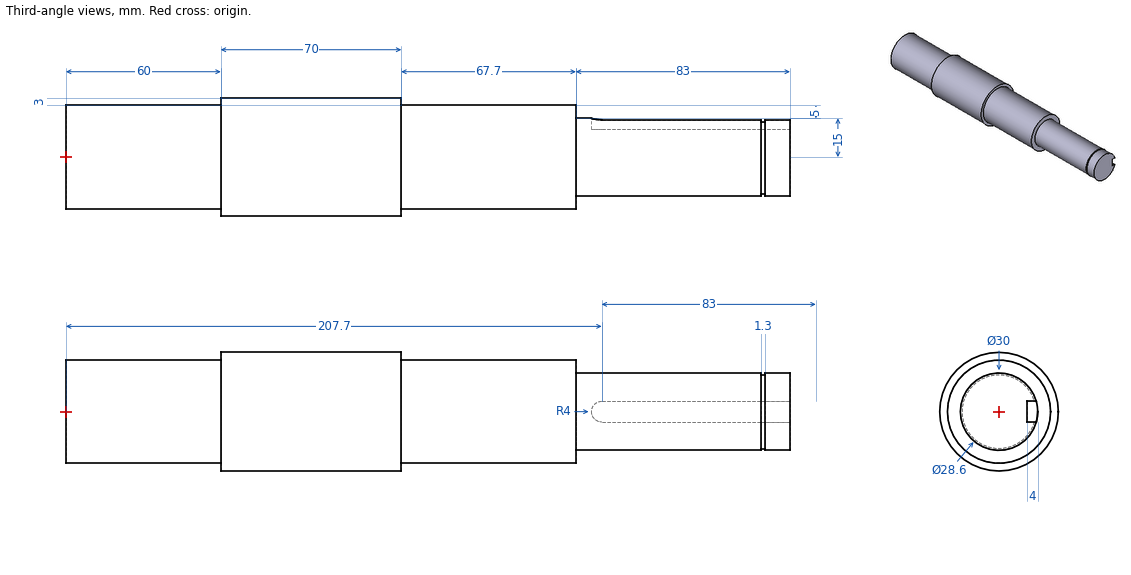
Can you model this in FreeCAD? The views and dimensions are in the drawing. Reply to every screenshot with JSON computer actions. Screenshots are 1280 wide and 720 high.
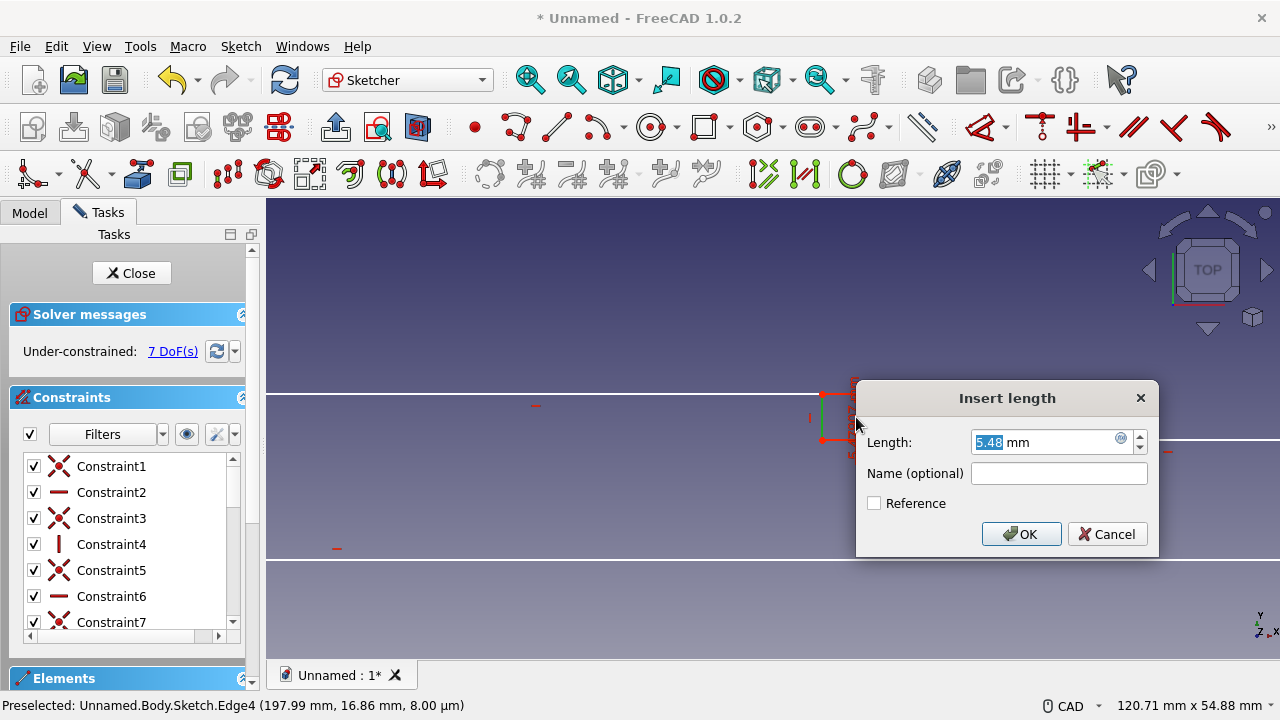
{"action": "type", "text": "5"}
{"action": "key", "text": "Return"}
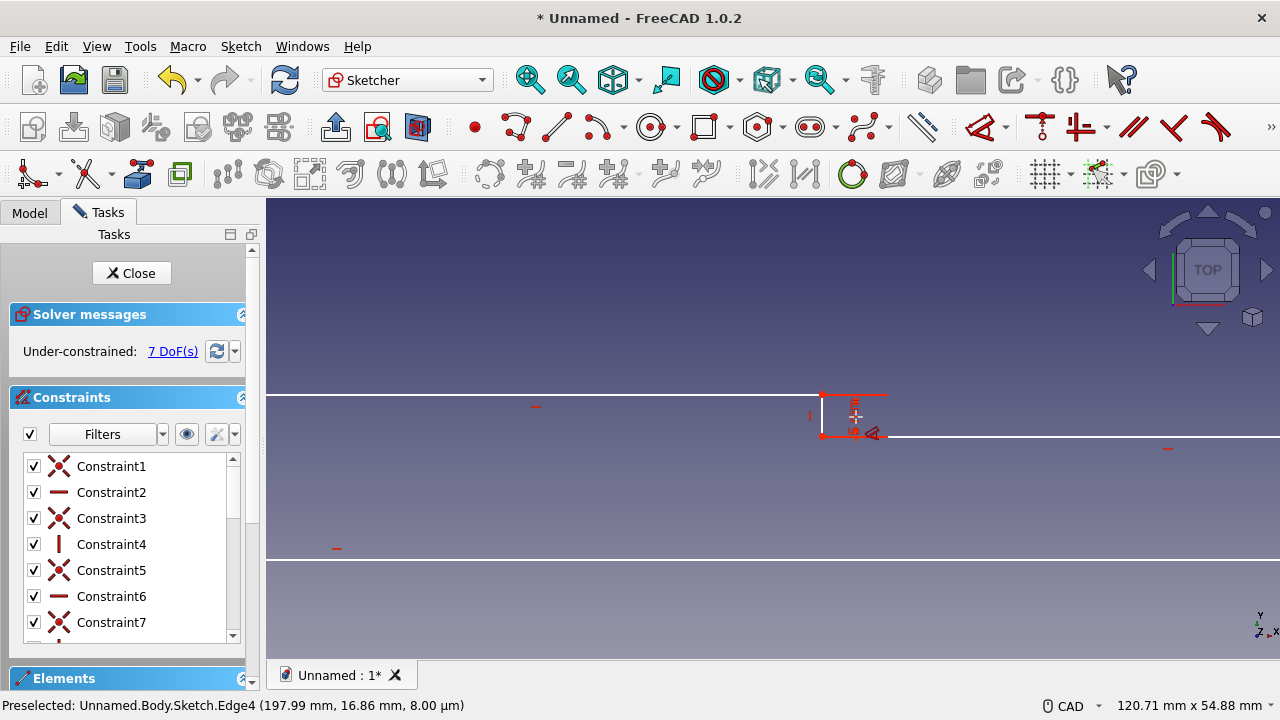
{"action": "scroll", "coordinate": [824, 417], "scroll_direction": "down", "scroll_amount": 7}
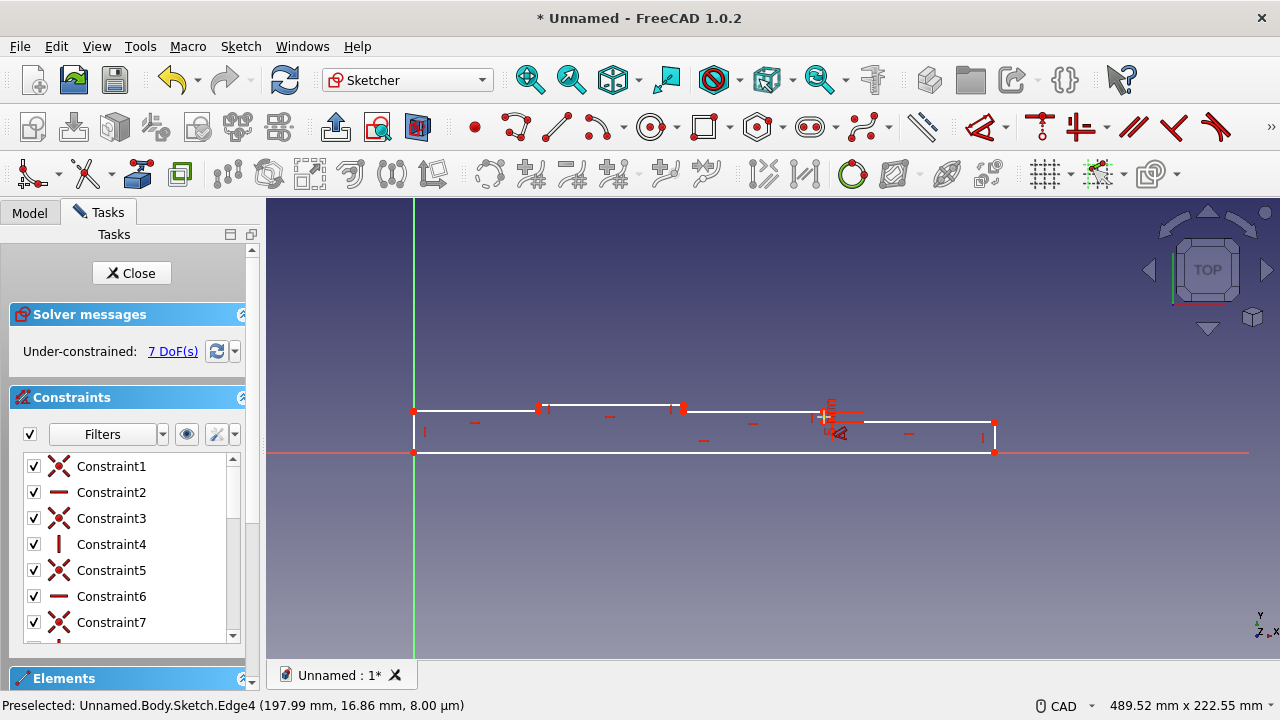
{"action": "scroll", "coordinate": [683, 409], "scroll_direction": "up", "scroll_amount": 10}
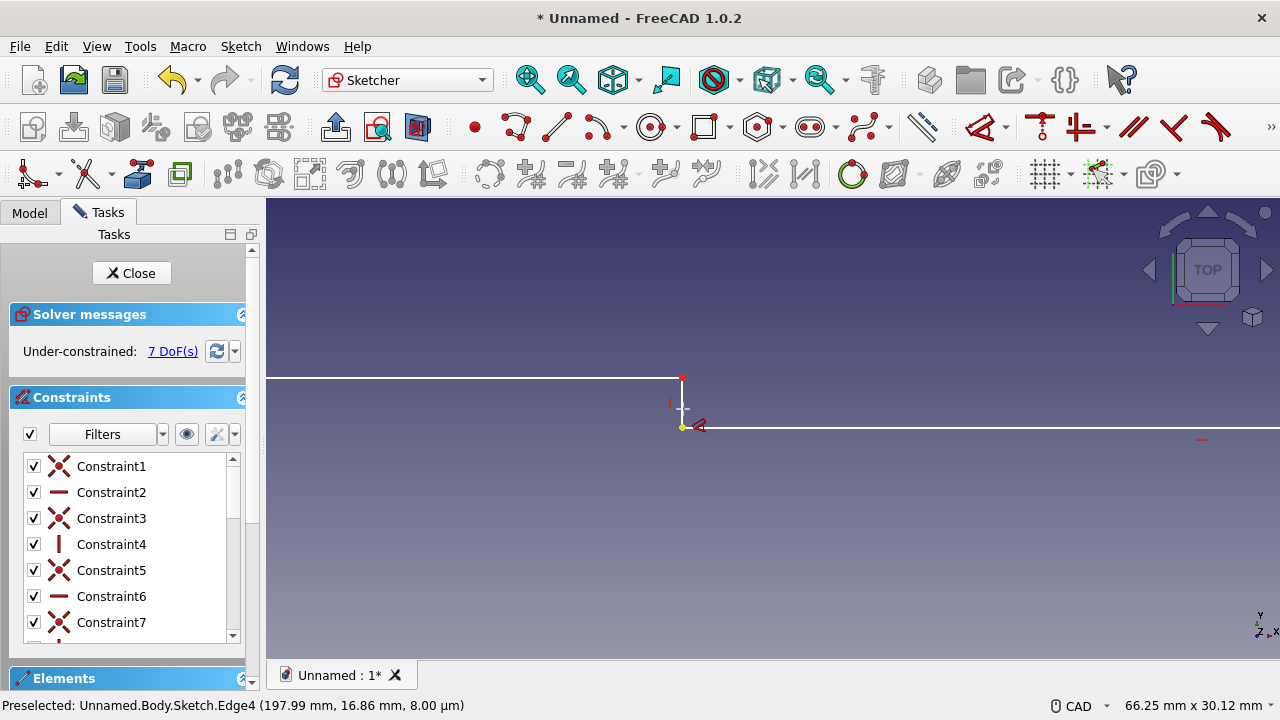
{"action": "left_click", "coordinate": [682, 408]}
{"action": "left_click", "coordinate": [648, 403]}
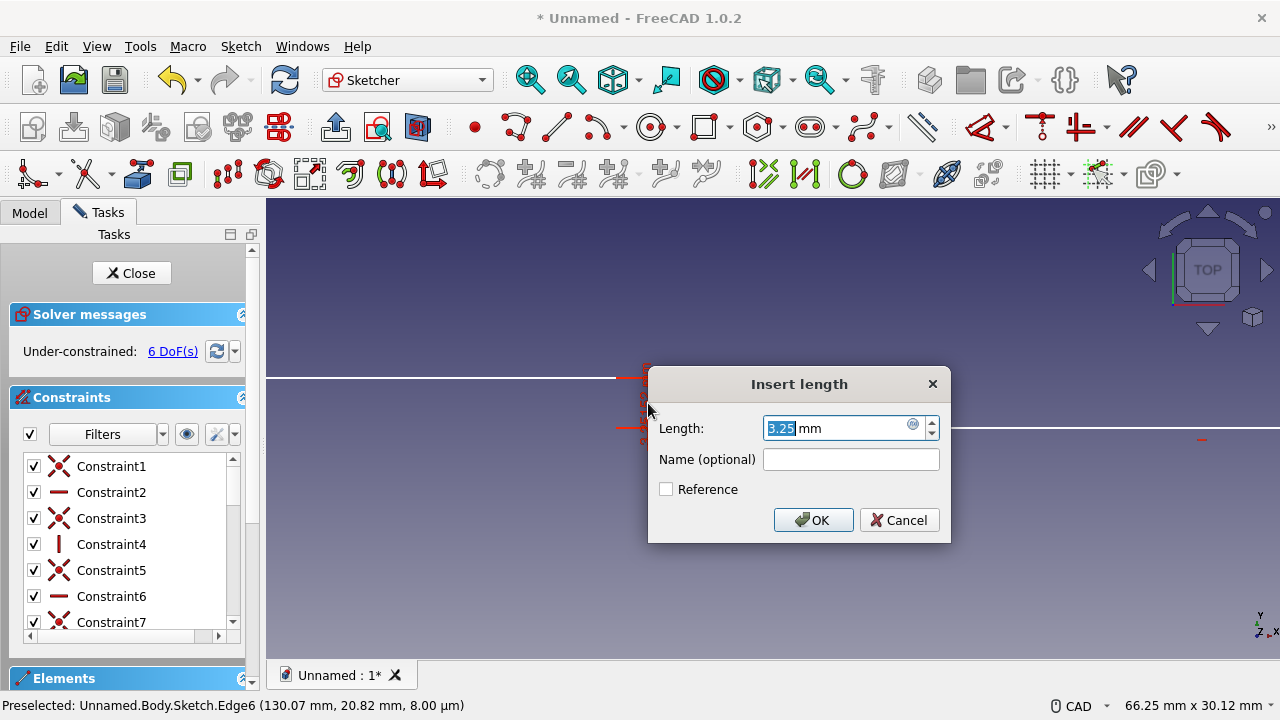
{"action": "type", "text": "3"}
{"action": "key", "text": "Return"}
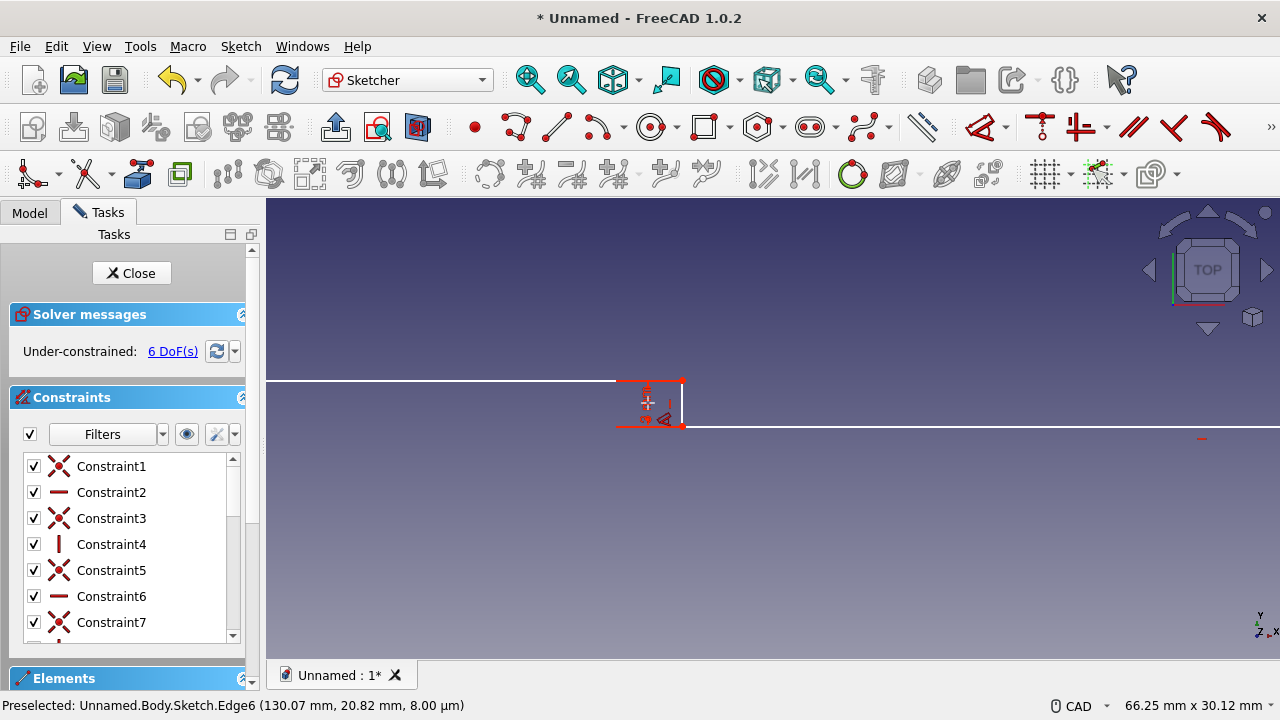
{"action": "scroll", "coordinate": [683, 409], "scroll_direction": "down", "scroll_amount": 10}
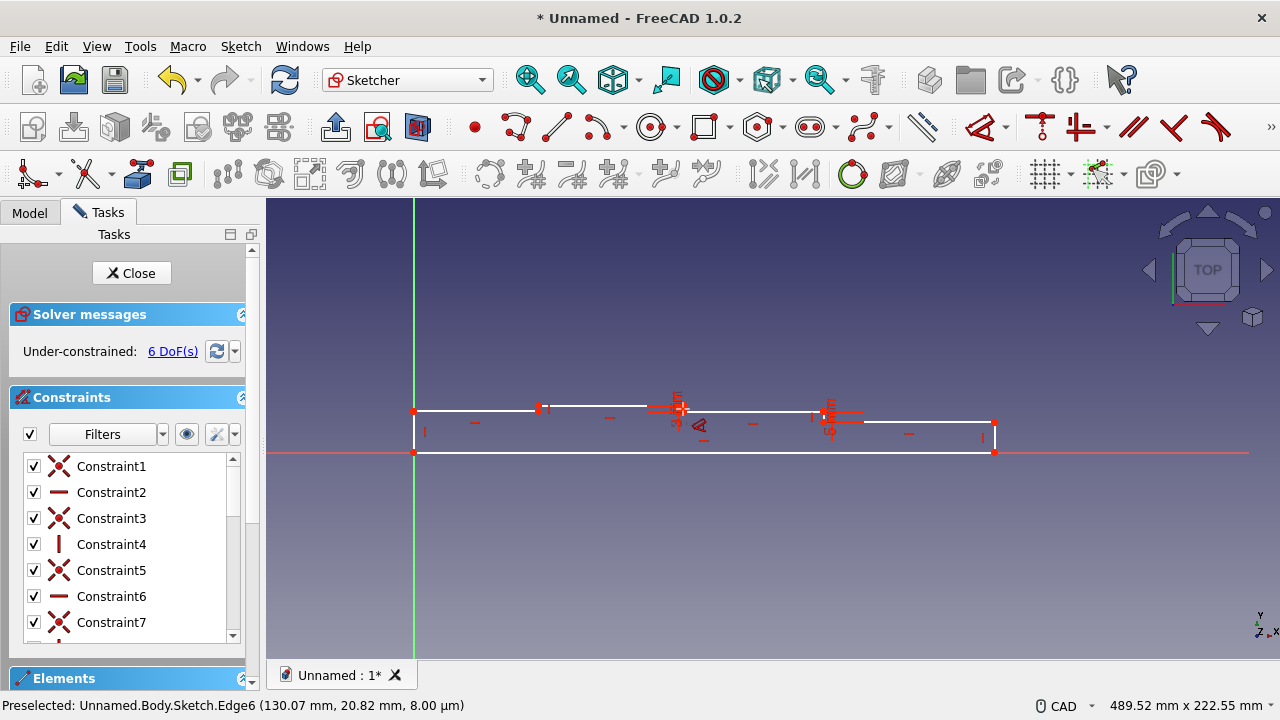
{"action": "scroll", "coordinate": [538, 407], "scroll_direction": "up", "scroll_amount": 11}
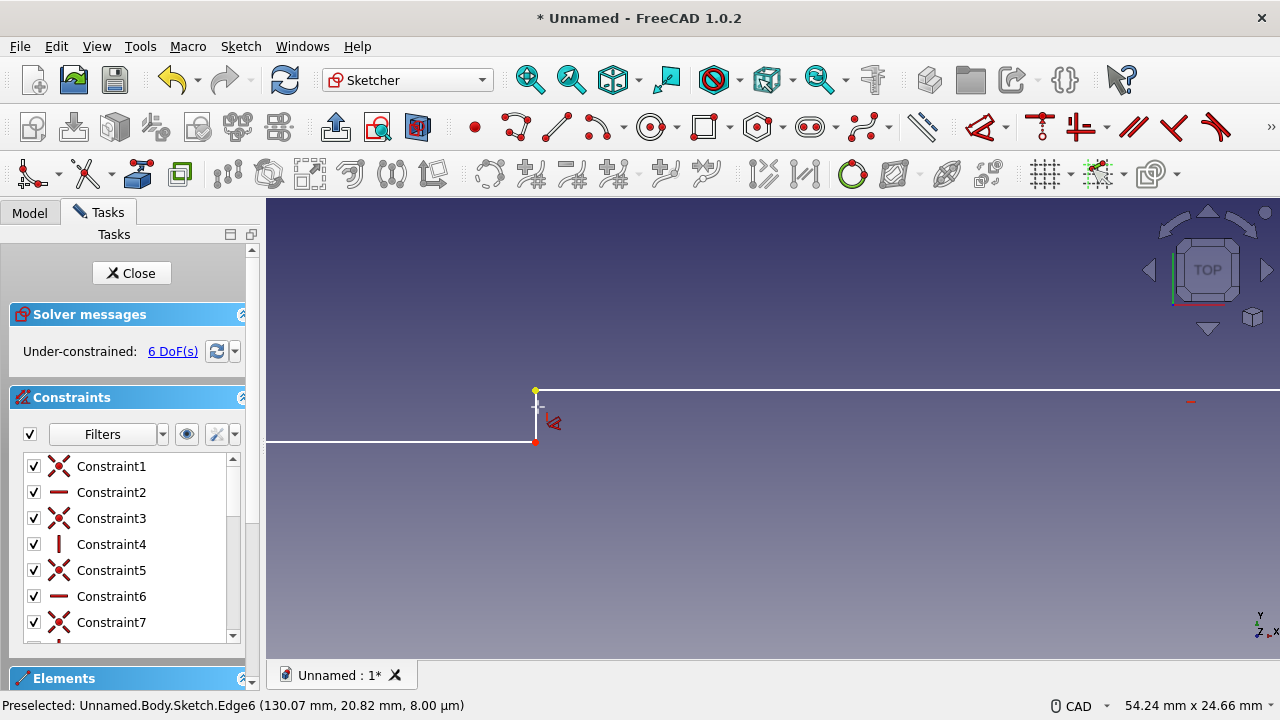
{"action": "left_click", "coordinate": [536, 406]}
{"action": "left_click", "coordinate": [502, 416]}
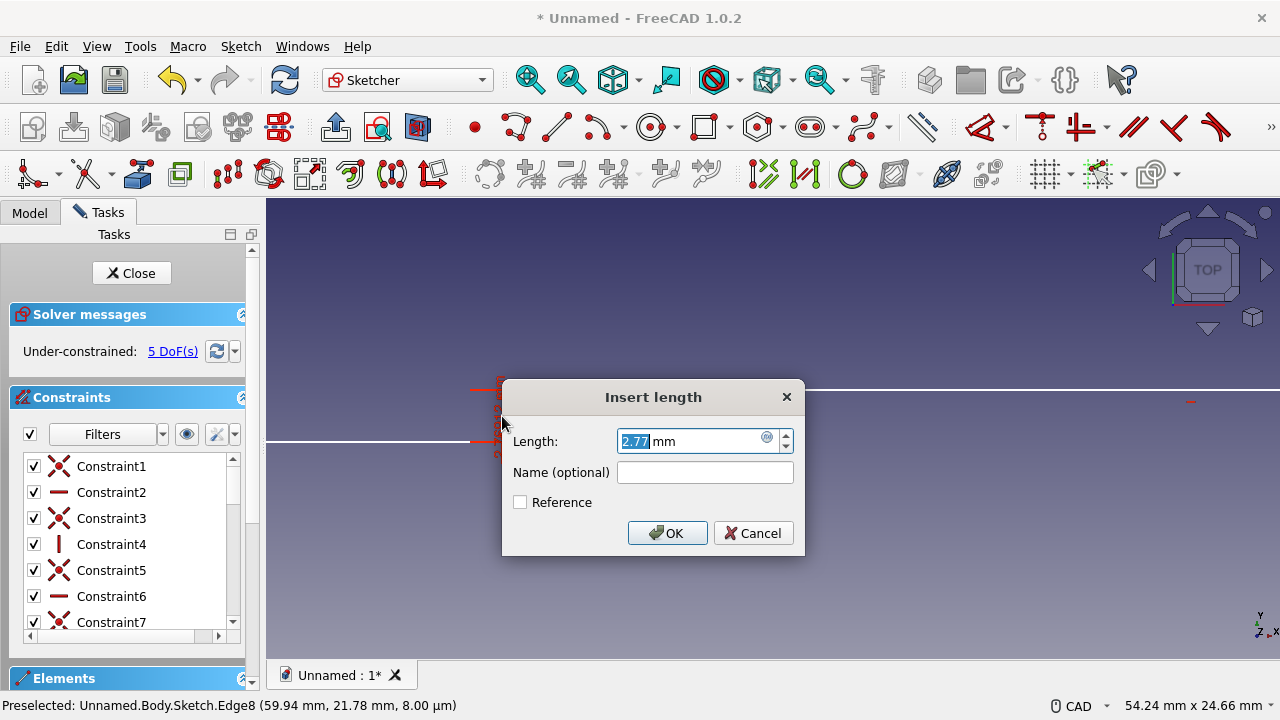
{"action": "type", "text": "3"}
{"action": "key", "text": "Return"}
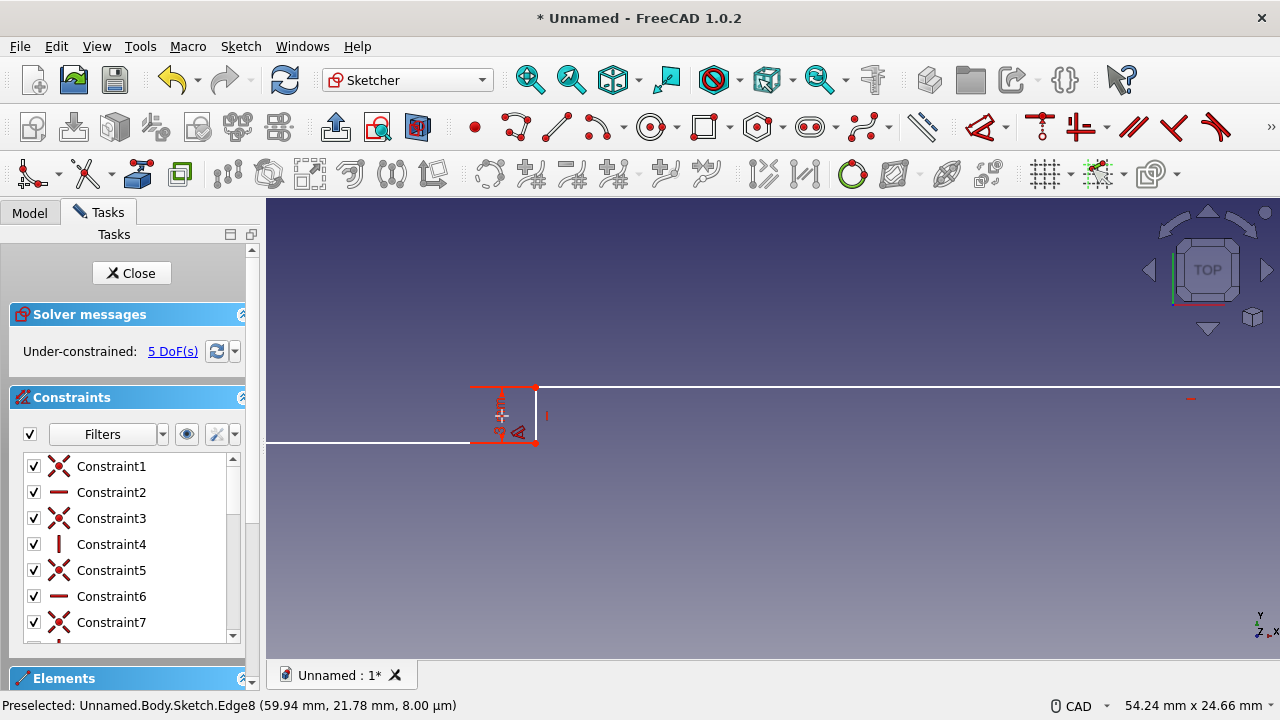
{"action": "scroll", "coordinate": [538, 407], "scroll_direction": "down", "scroll_amount": 11}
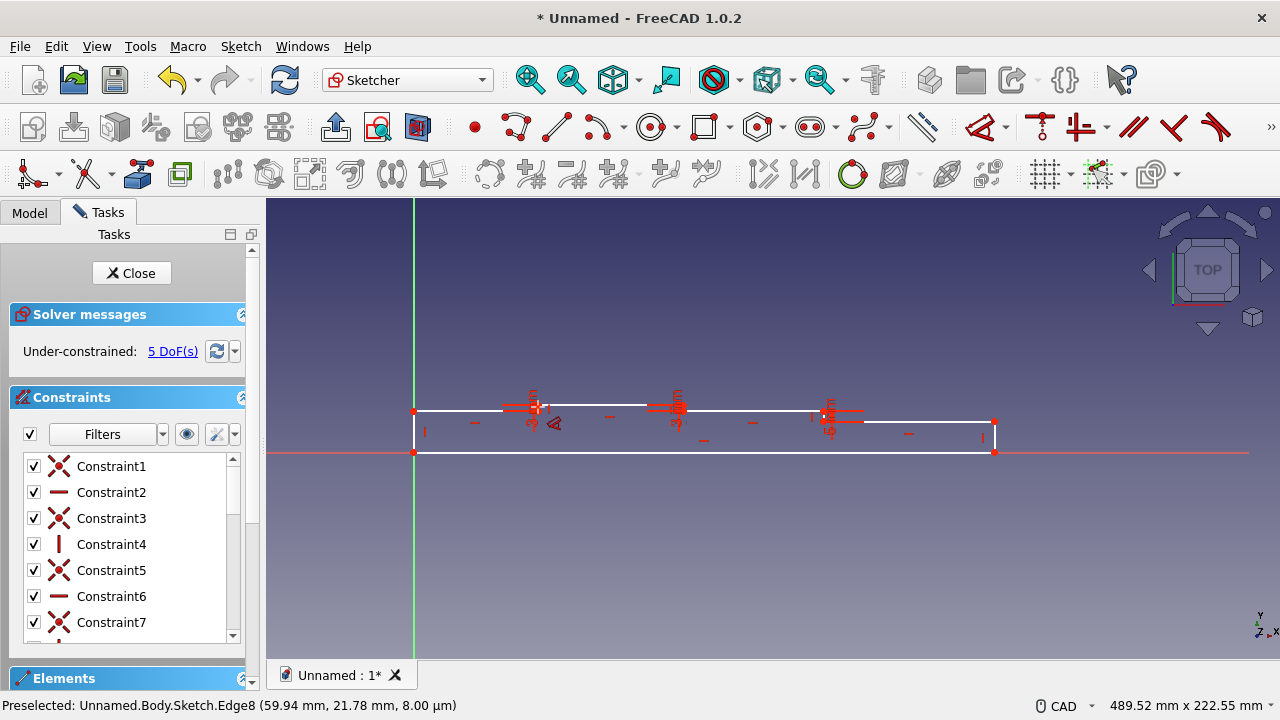
{"action": "scroll", "coordinate": [995, 443], "scroll_direction": "up", "scroll_amount": 3}